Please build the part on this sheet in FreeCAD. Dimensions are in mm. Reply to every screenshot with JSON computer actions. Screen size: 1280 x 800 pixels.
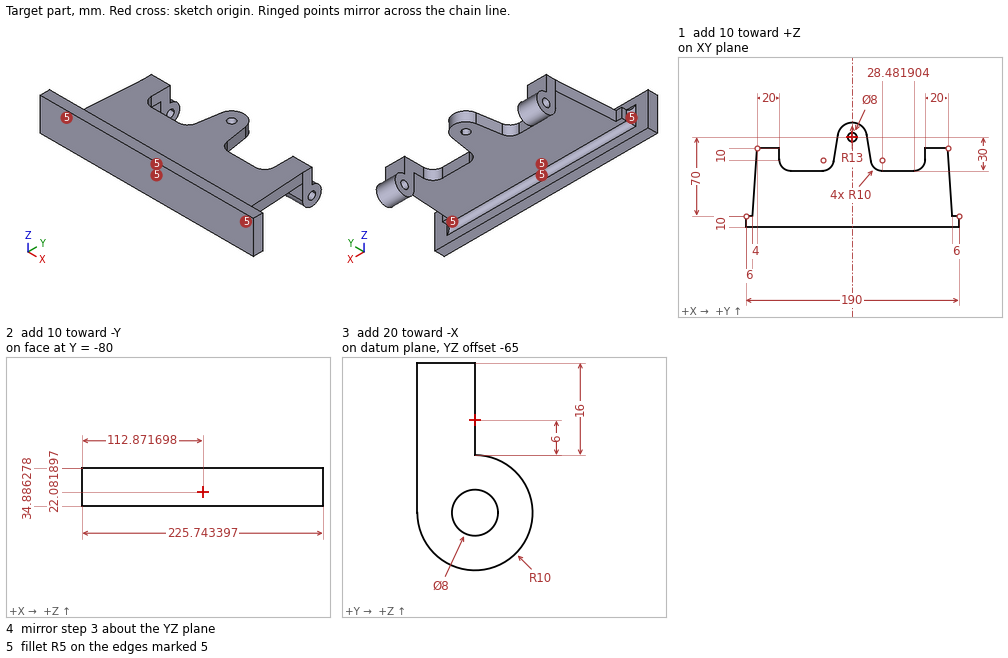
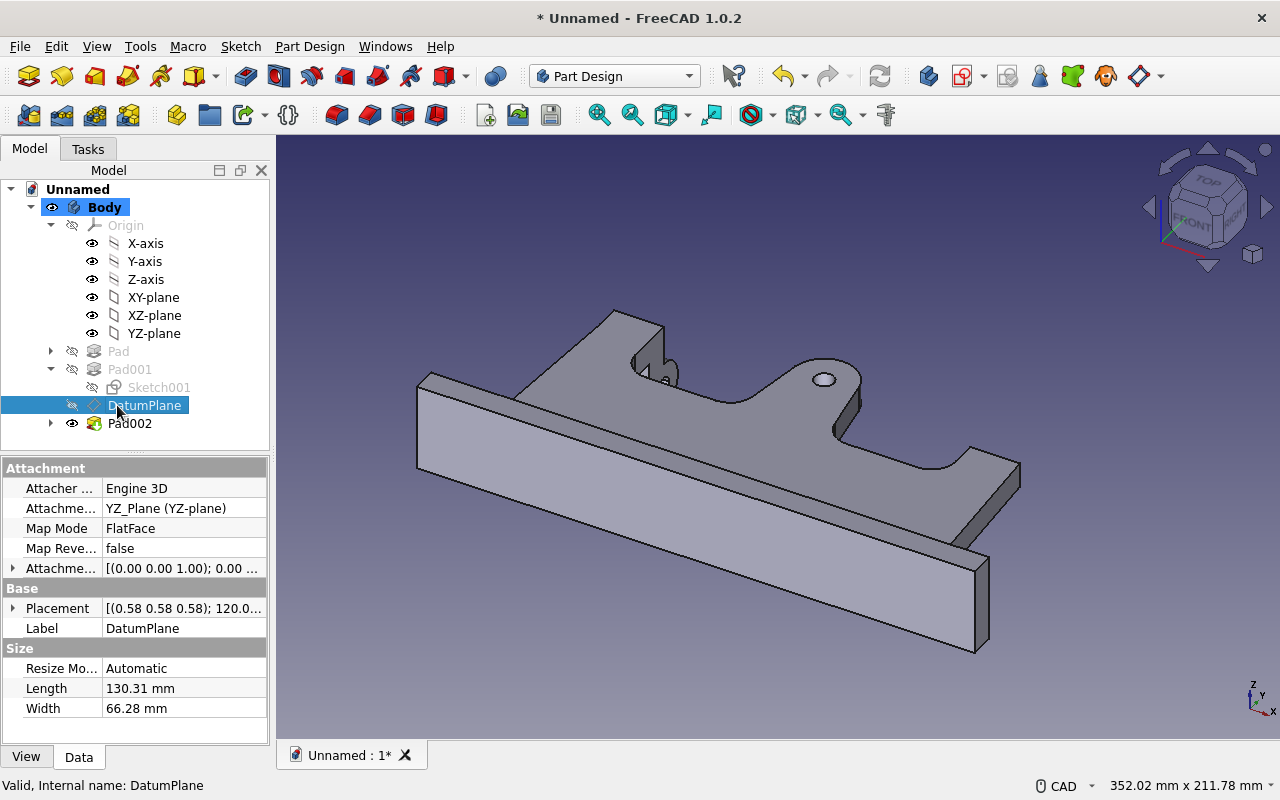
{"action": "left_click", "coordinate": [117, 423]}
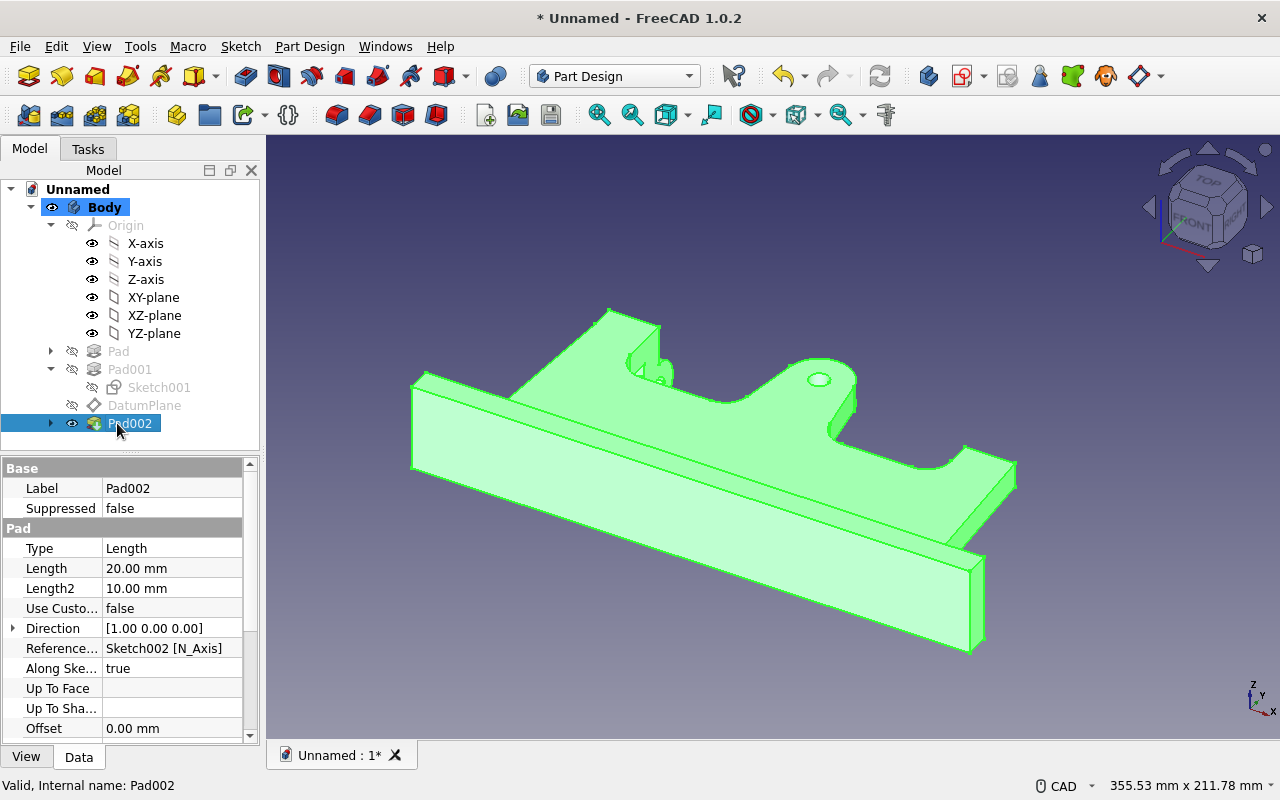
{"action": "left_click", "coordinate": [29, 116]}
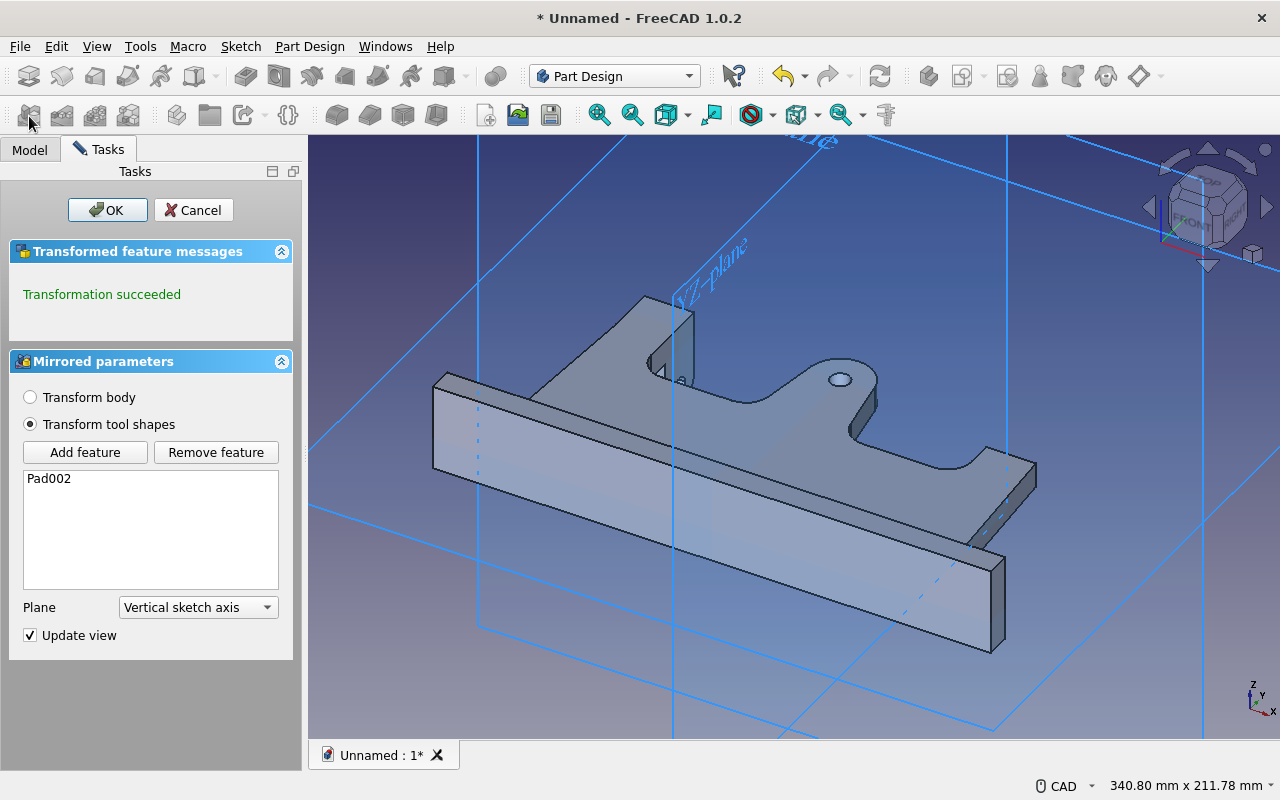
{"action": "left_click", "coordinate": [199, 608]}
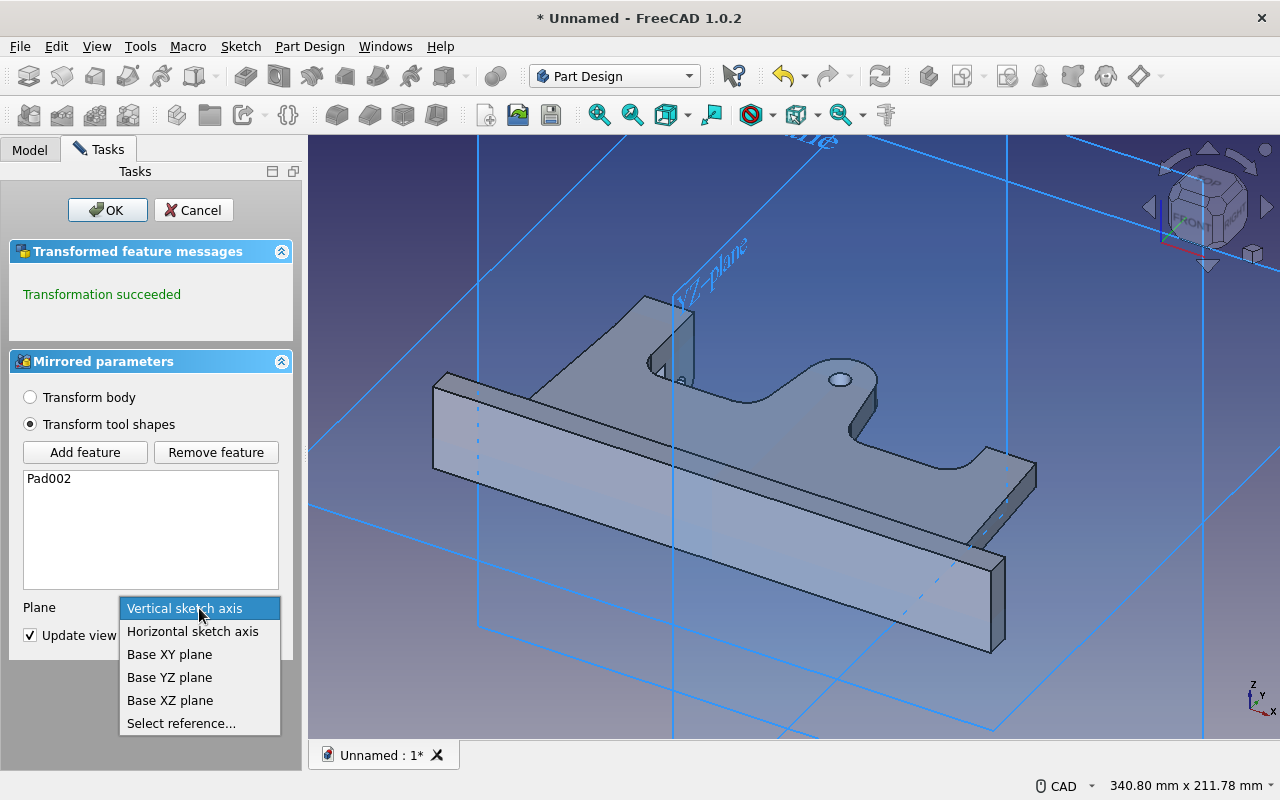
{"action": "left_click", "coordinate": [198, 678]}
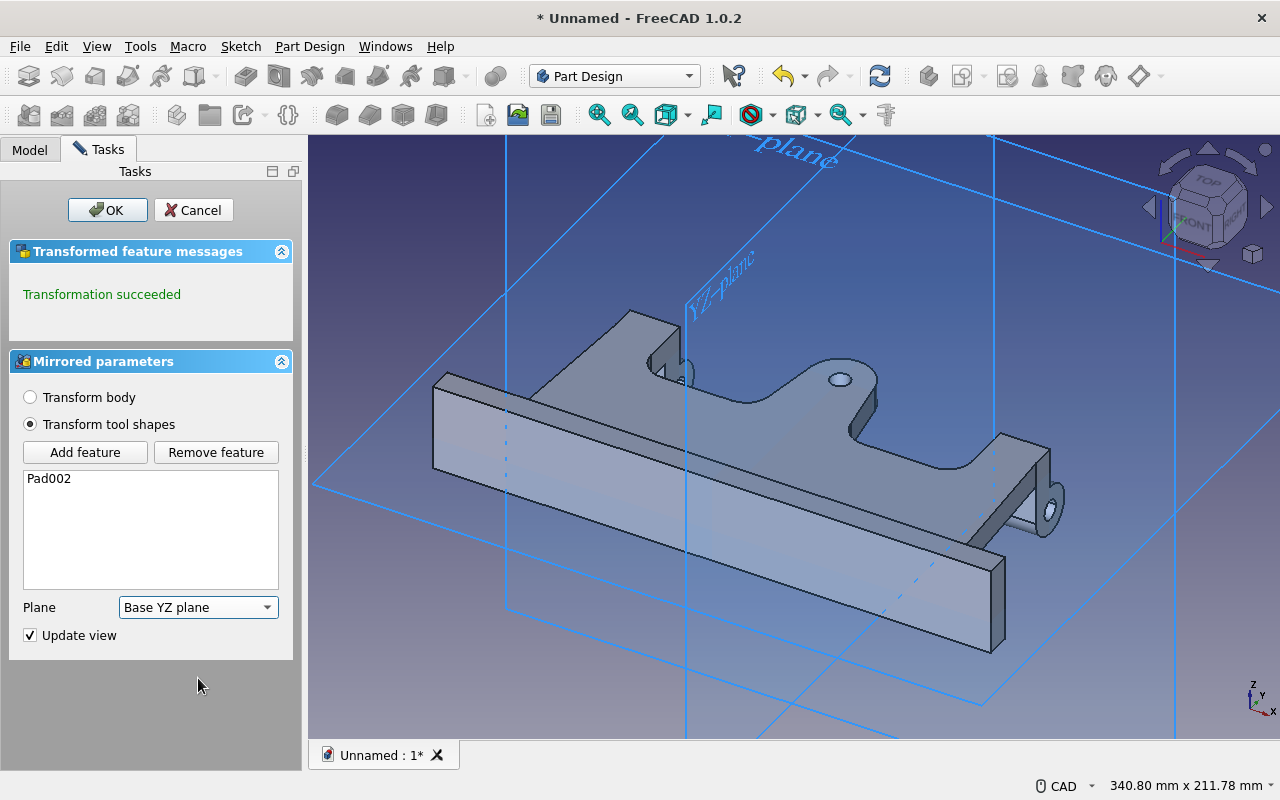
{"action": "left_click", "coordinate": [108, 210]}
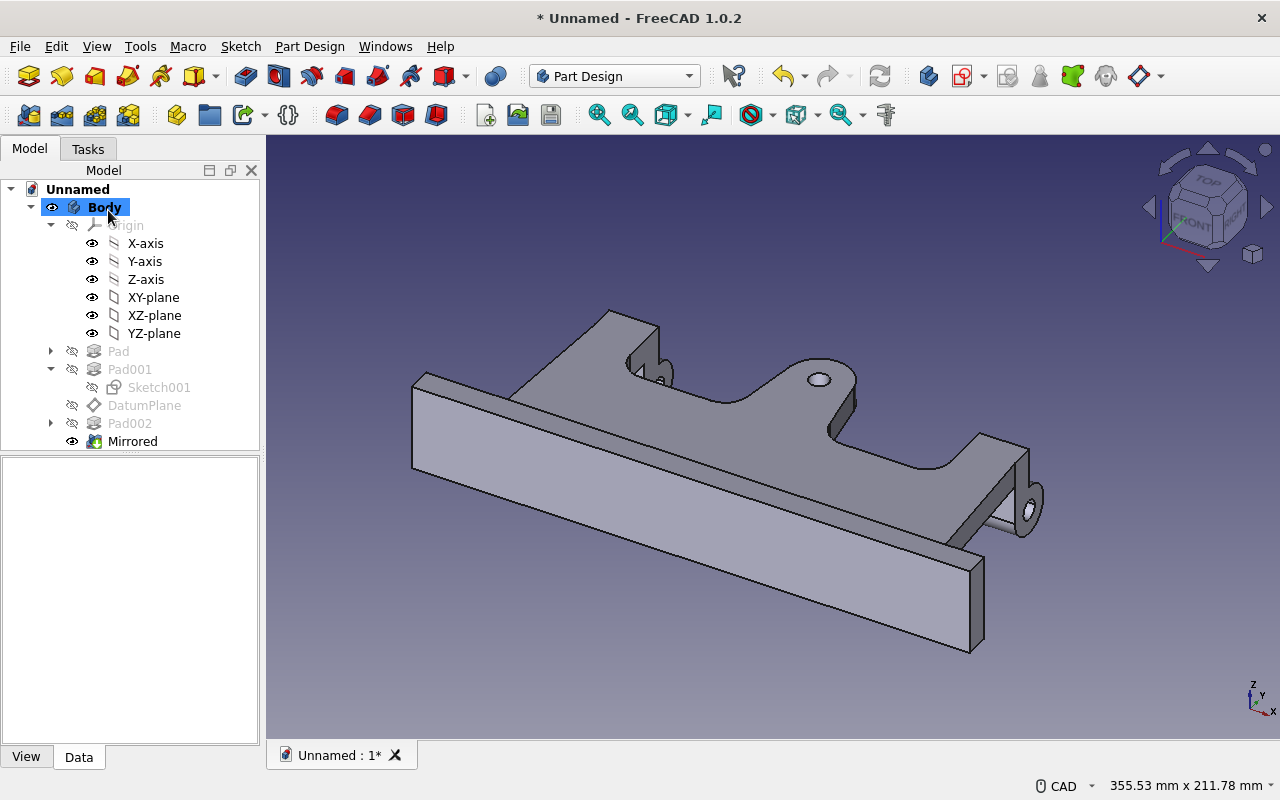
{"action": "key", "text": "0"}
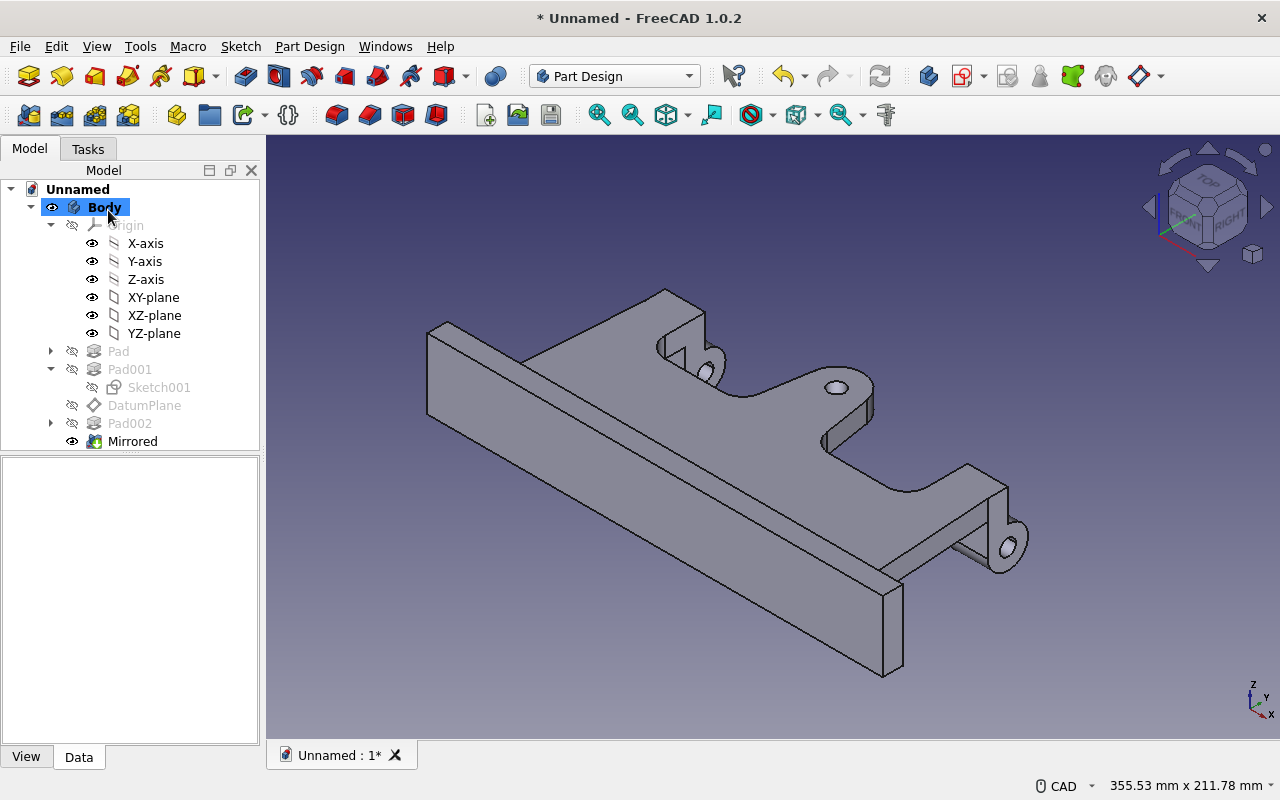
{"action": "key", "text": "2"}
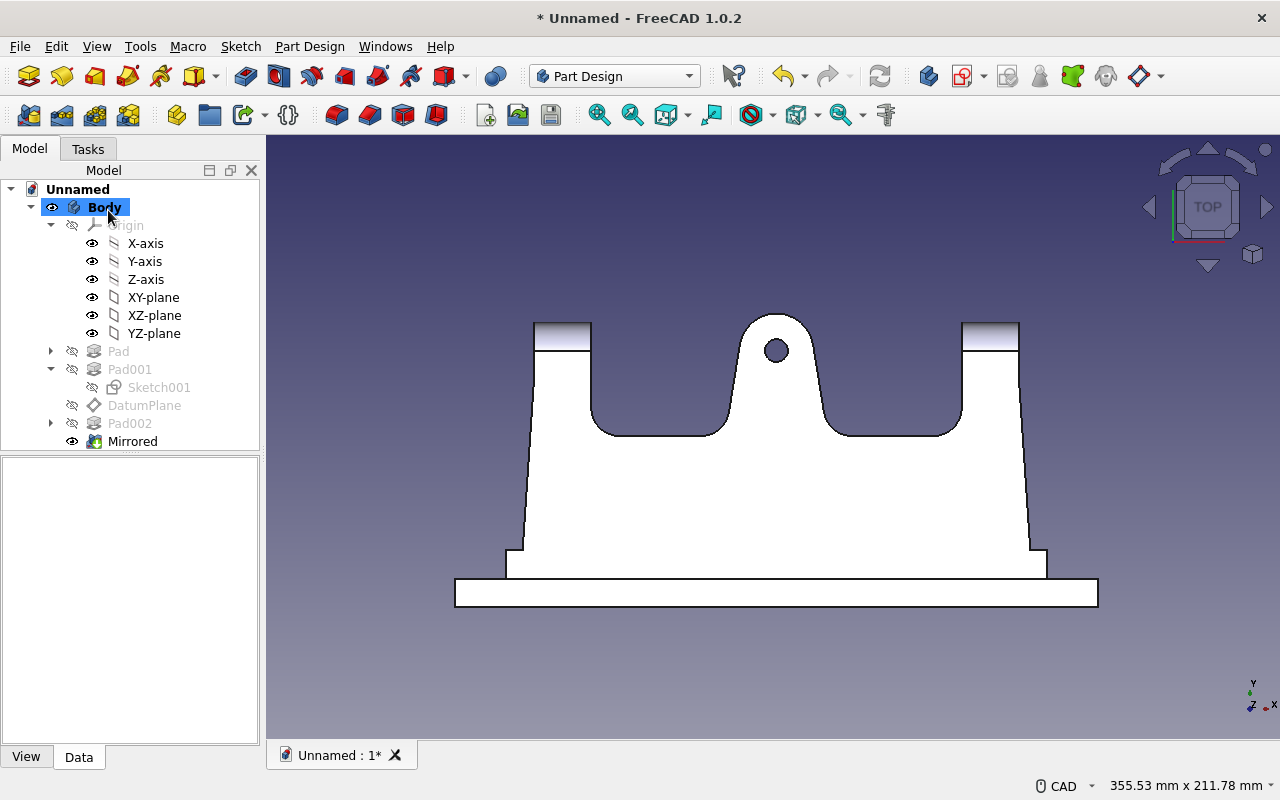
{"action": "key", "text": "1"}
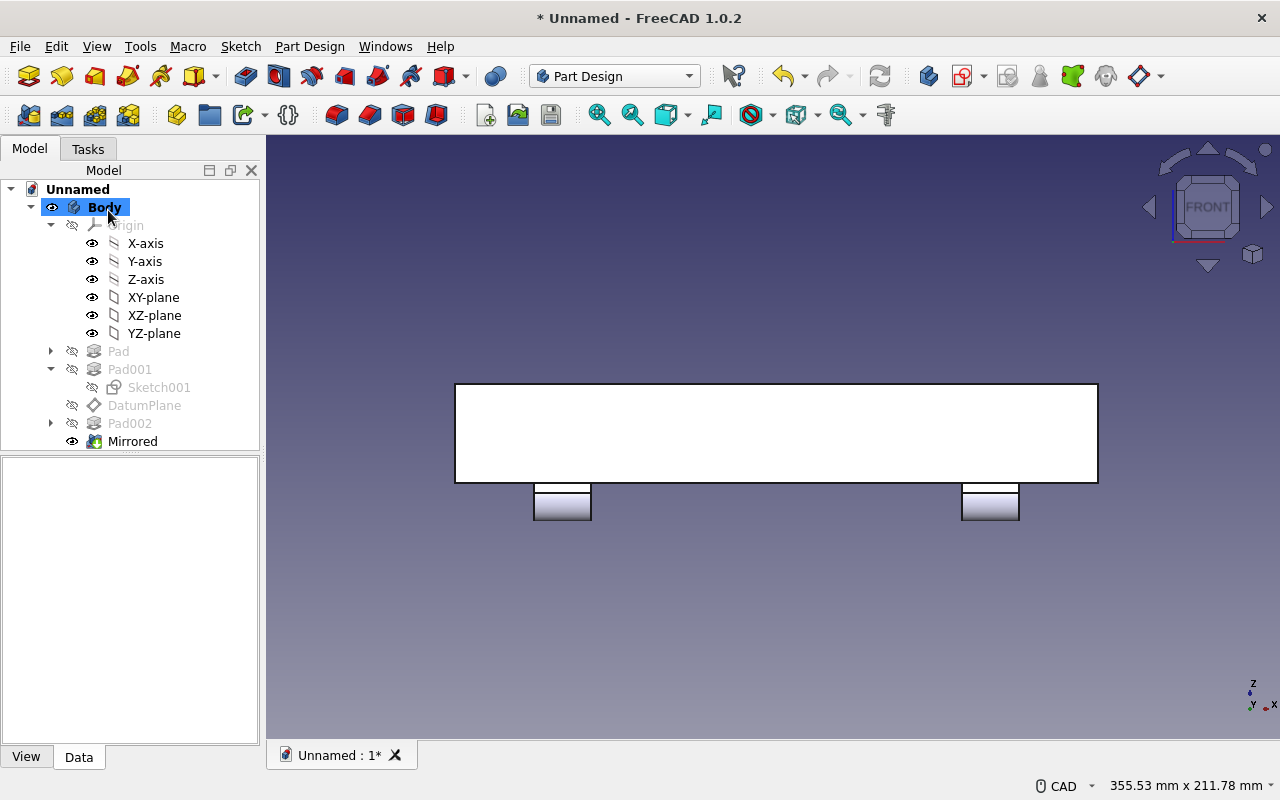
{"action": "key", "text": "3"}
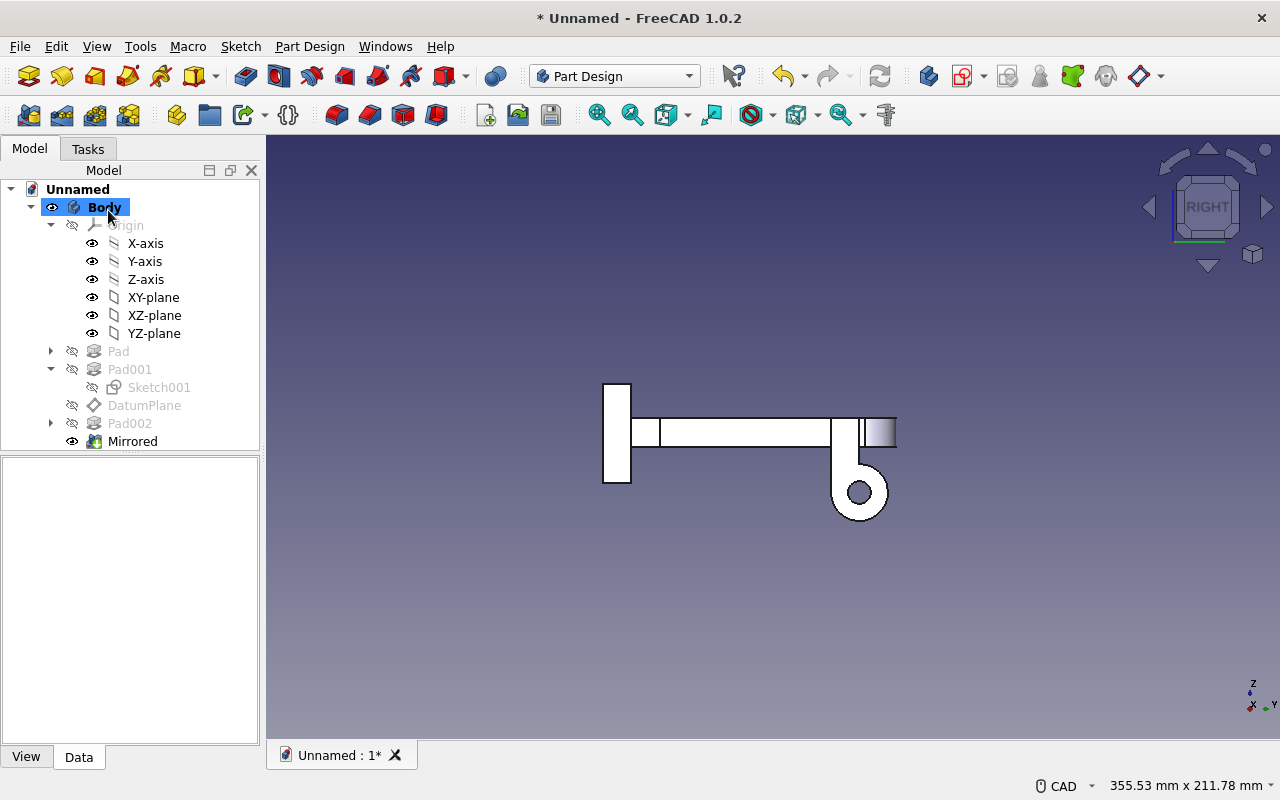
{"action": "left_click", "coordinate": [600, 116]}